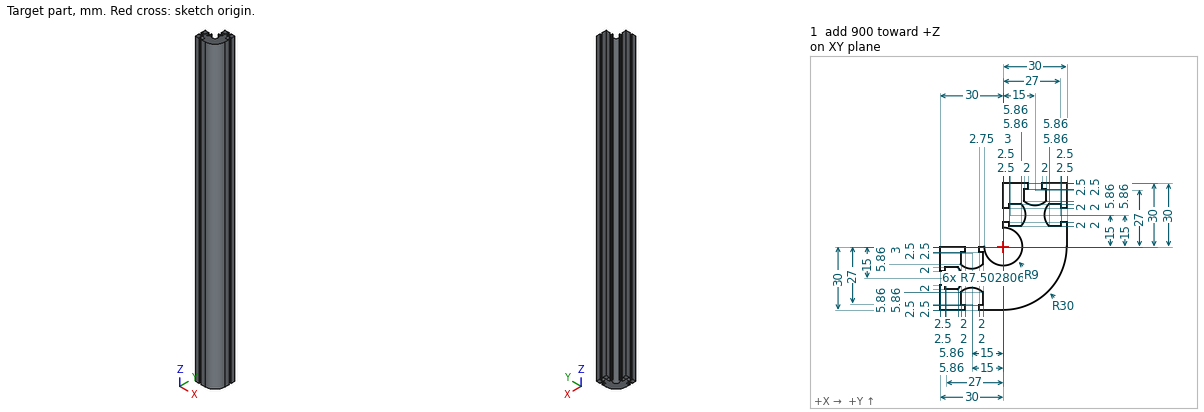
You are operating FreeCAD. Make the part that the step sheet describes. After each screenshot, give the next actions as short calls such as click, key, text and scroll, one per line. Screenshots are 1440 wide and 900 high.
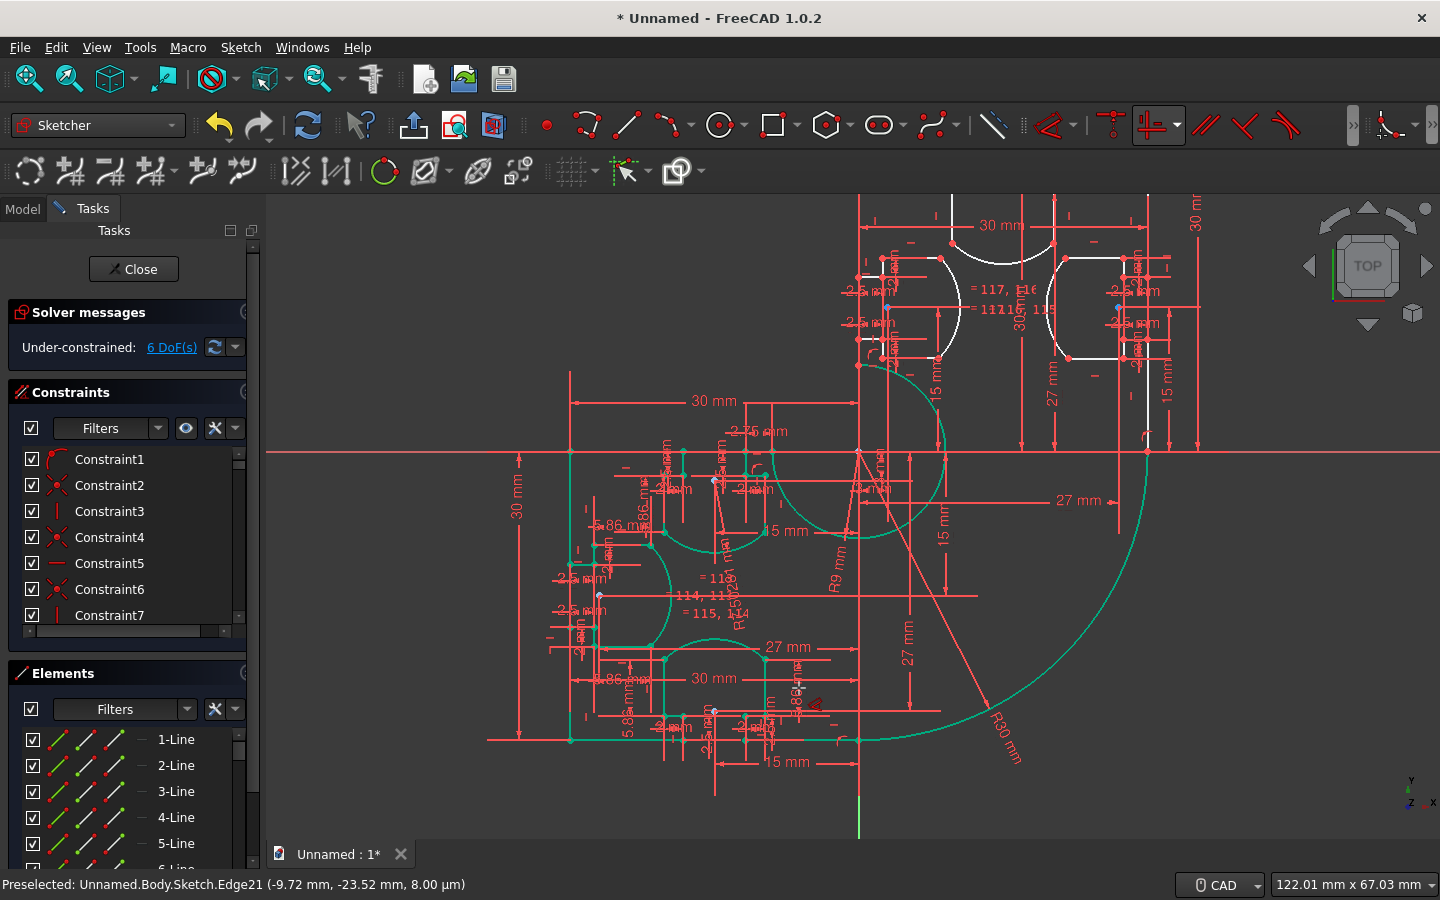
click(1107, 359)
click(1096, 417)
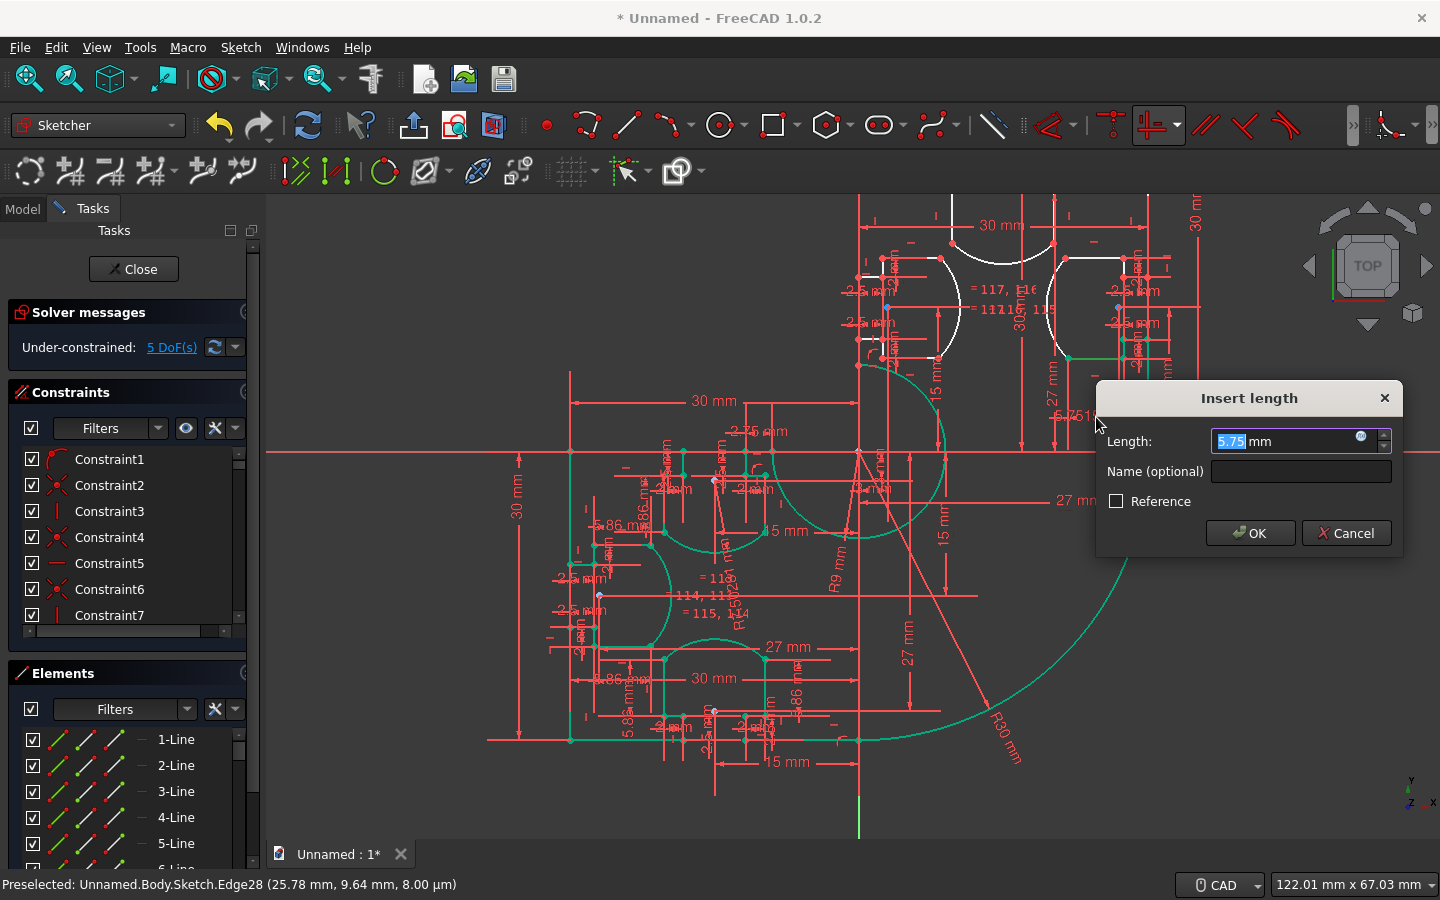
text(5.86)
key(Return)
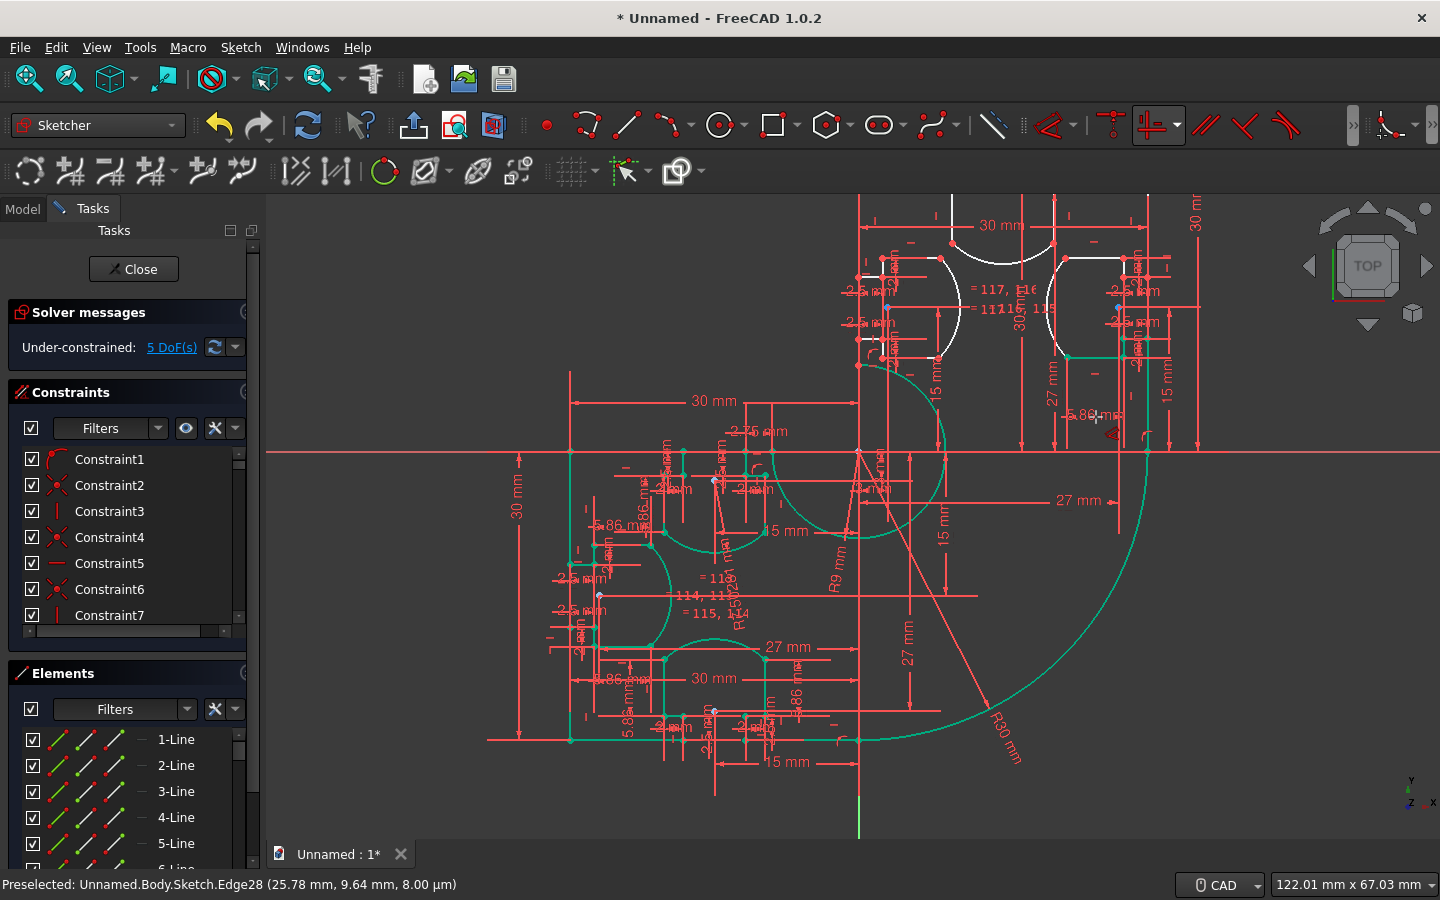
click(1083, 258)
click(1095, 224)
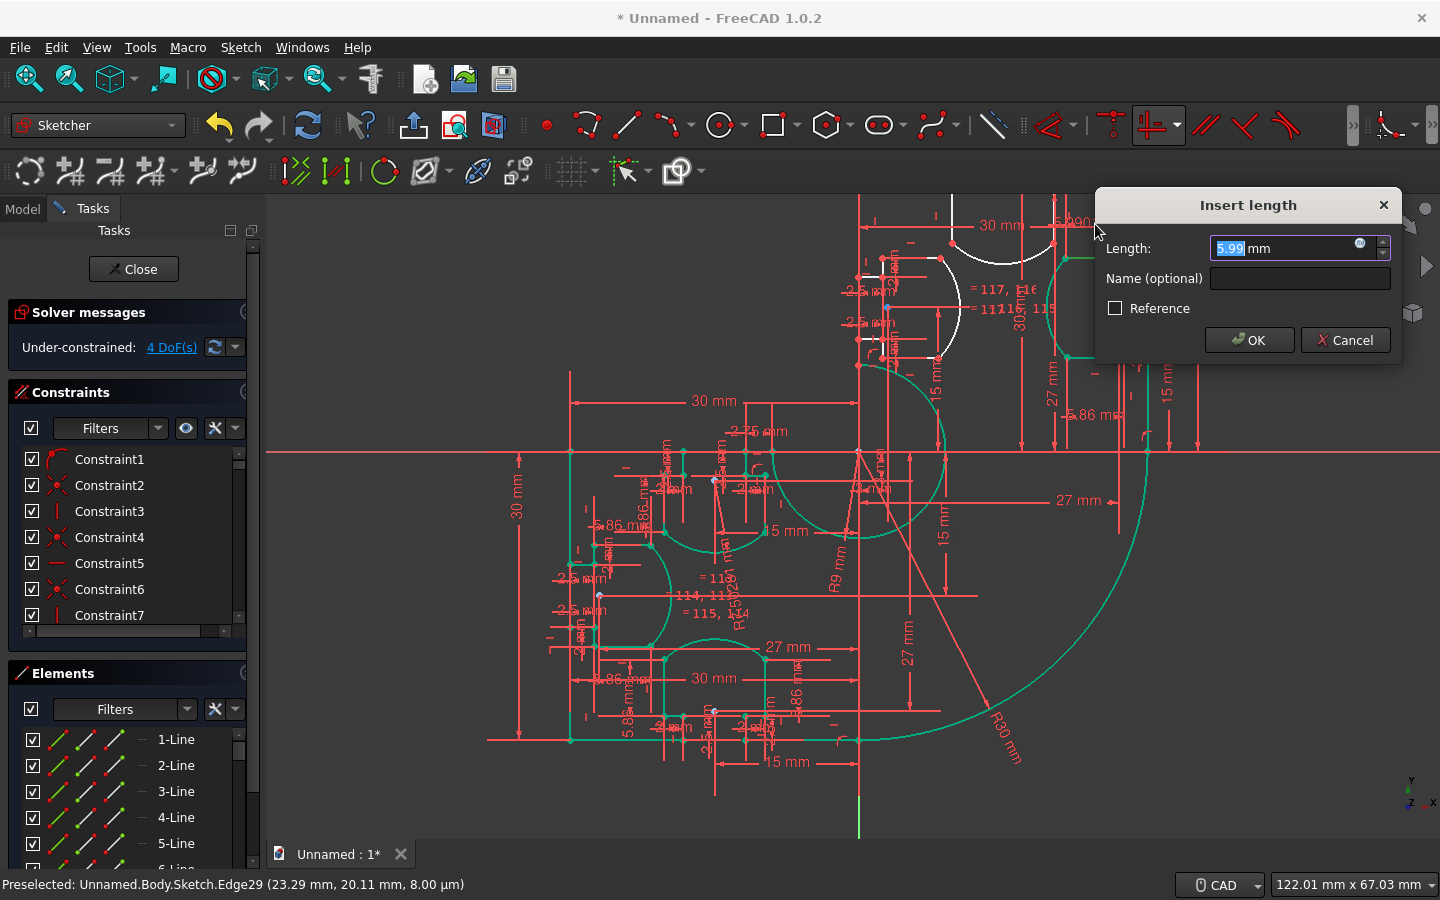
text(5.86)
key(Return)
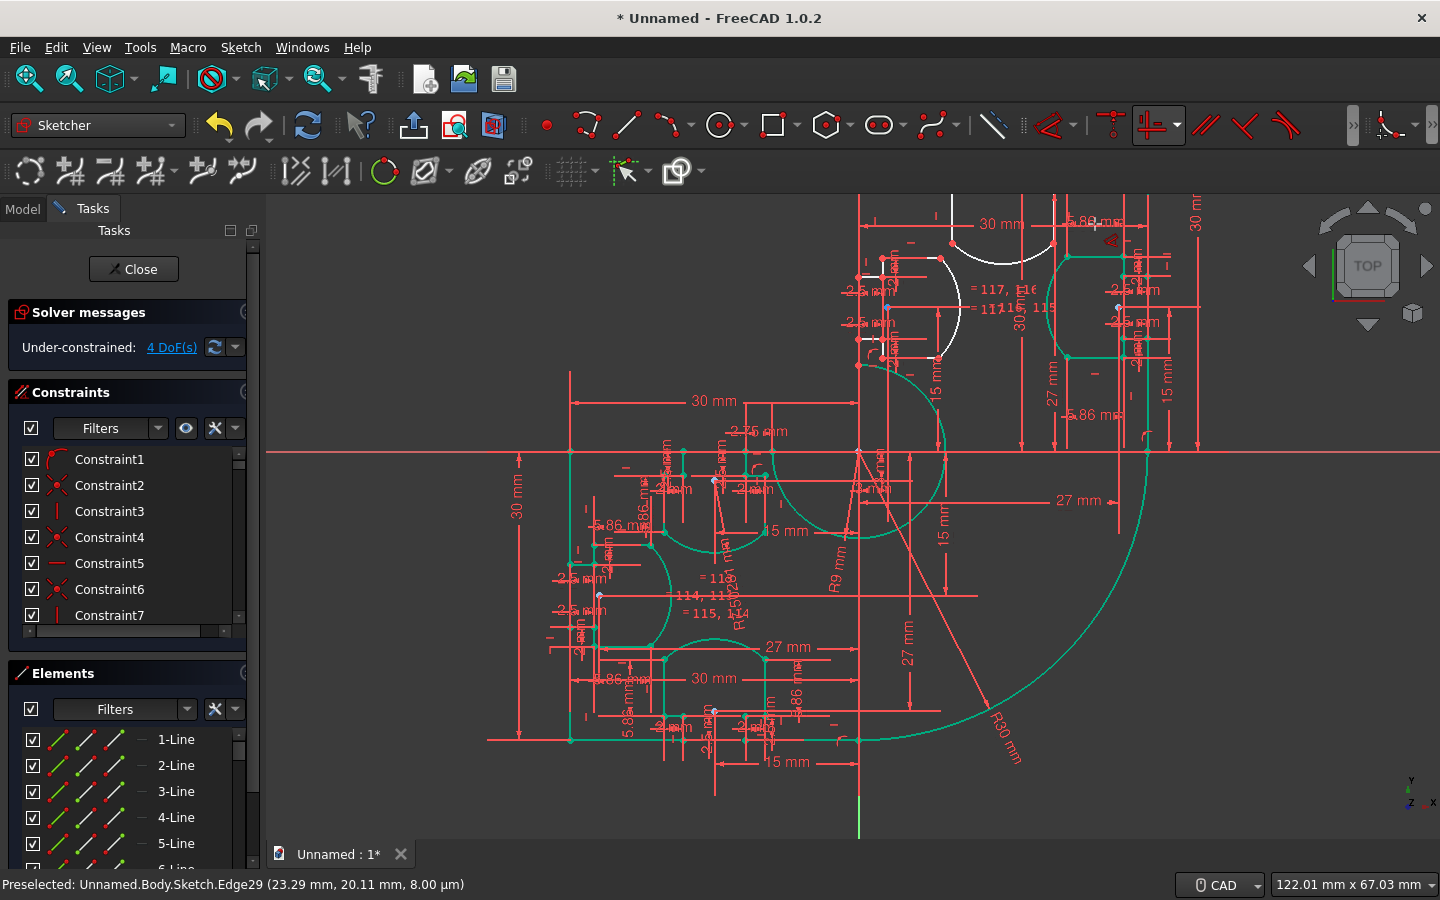
click(1054, 227)
click(1184, 233)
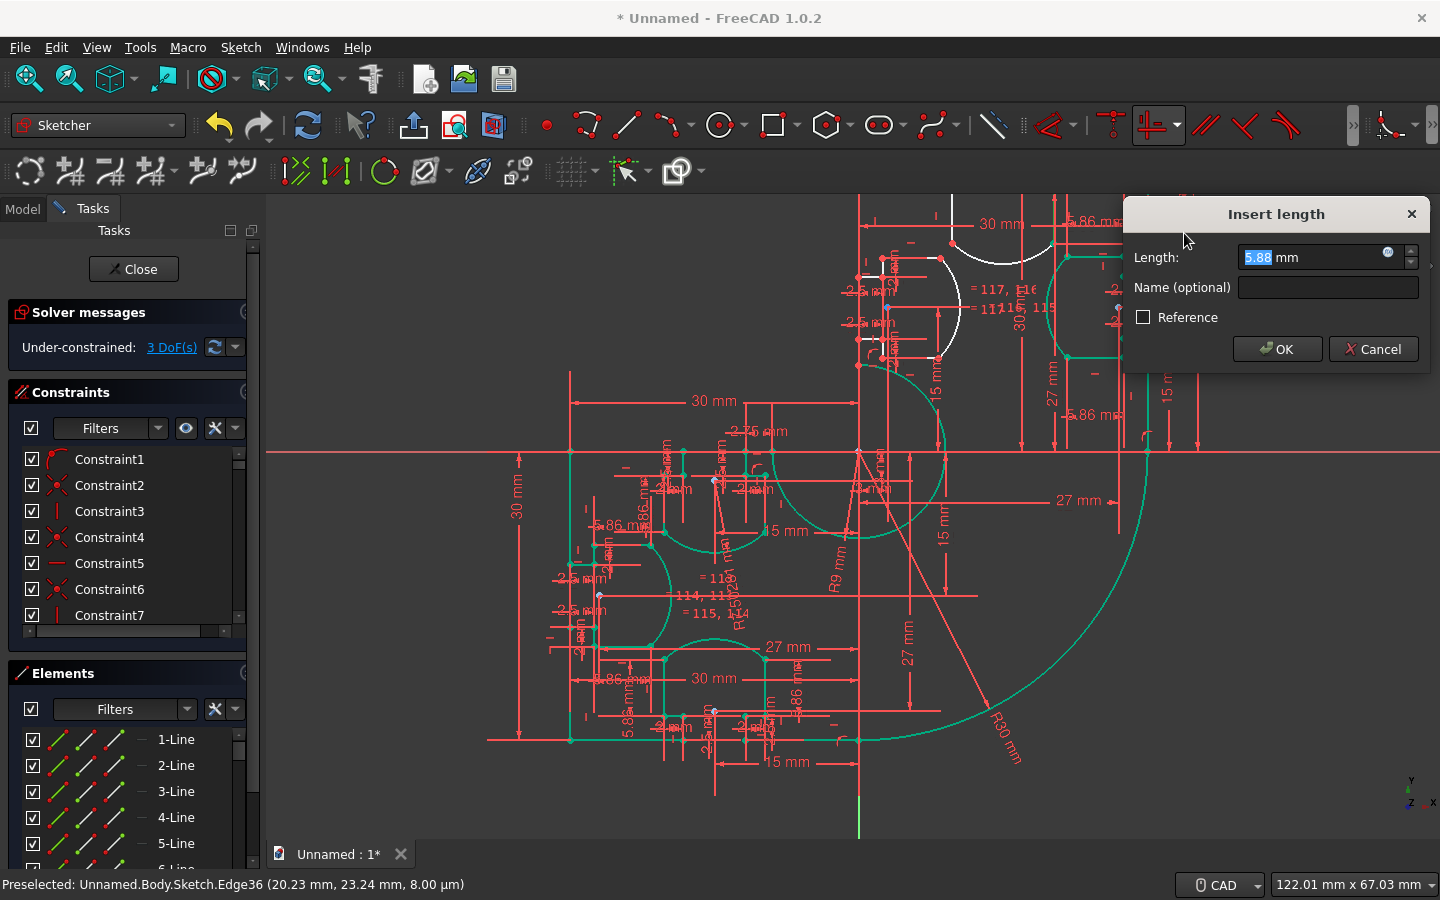
text(5.86)
key(Return)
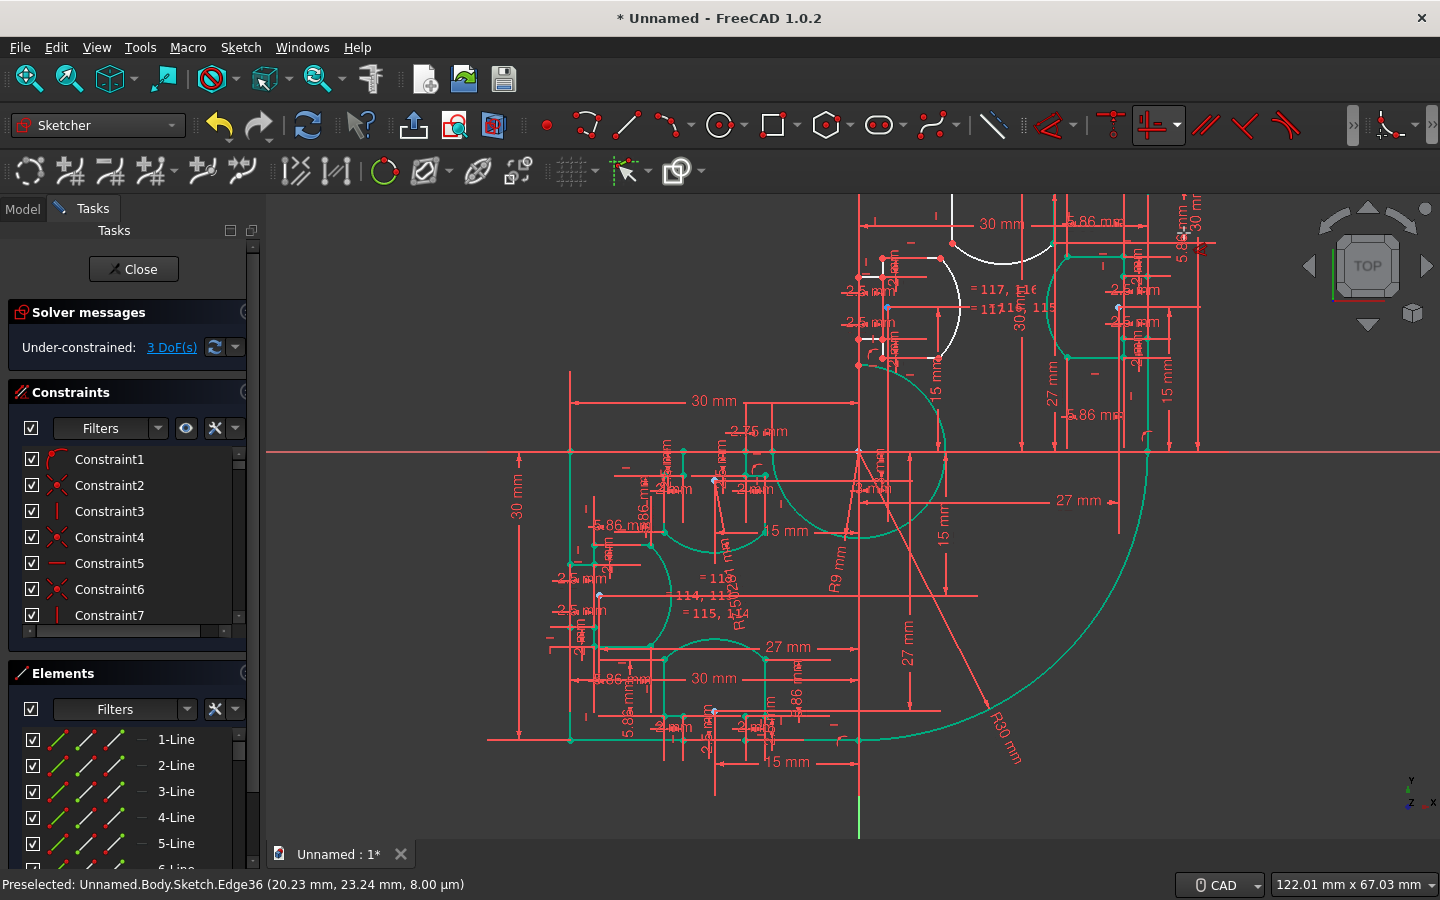
click(952, 226)
click(918, 233)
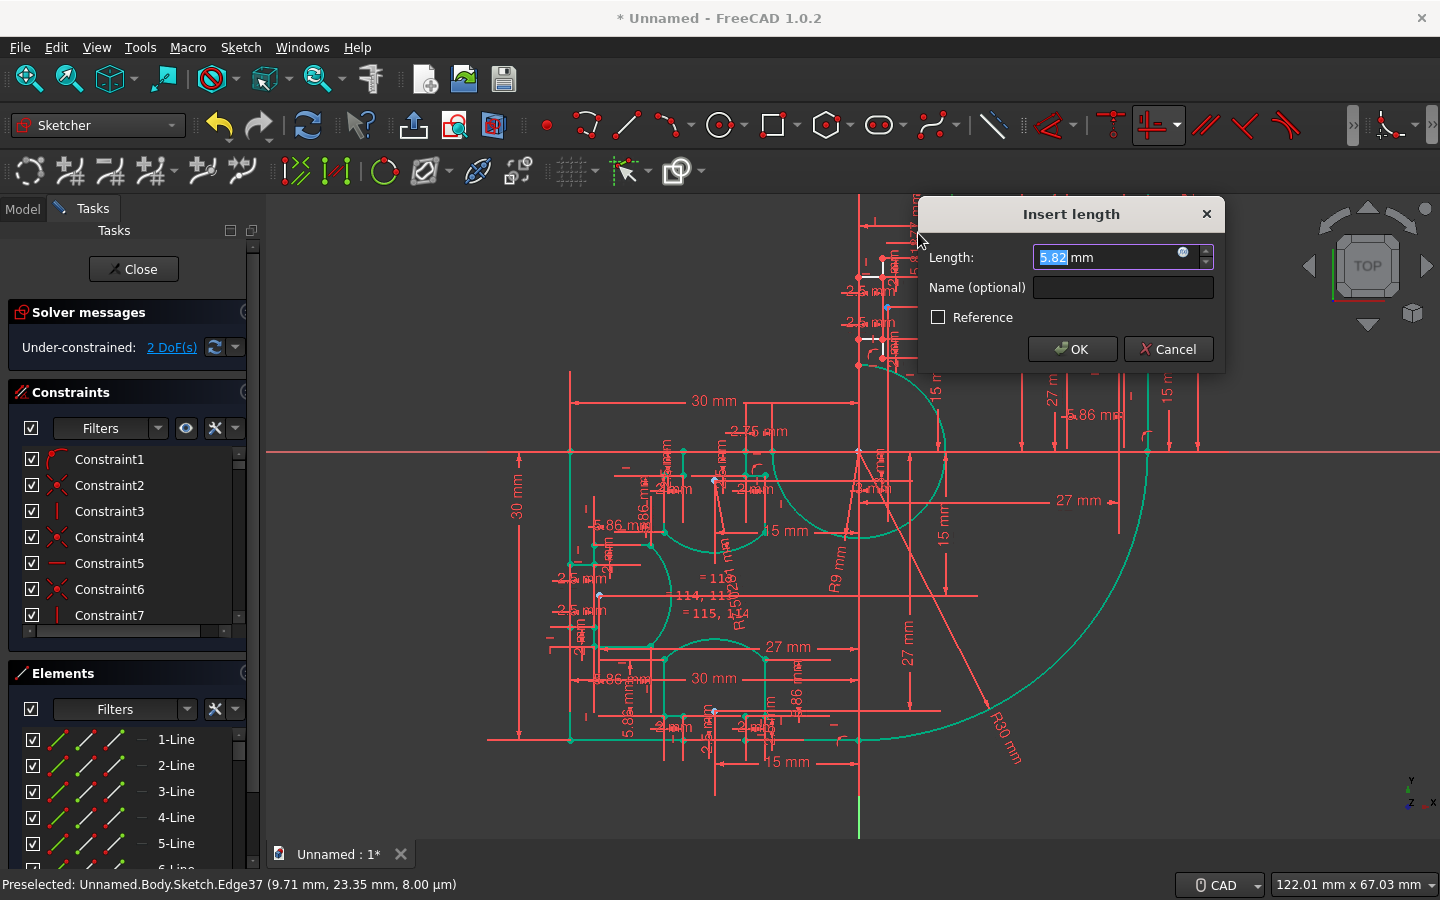
text(5.86)
key(Return)